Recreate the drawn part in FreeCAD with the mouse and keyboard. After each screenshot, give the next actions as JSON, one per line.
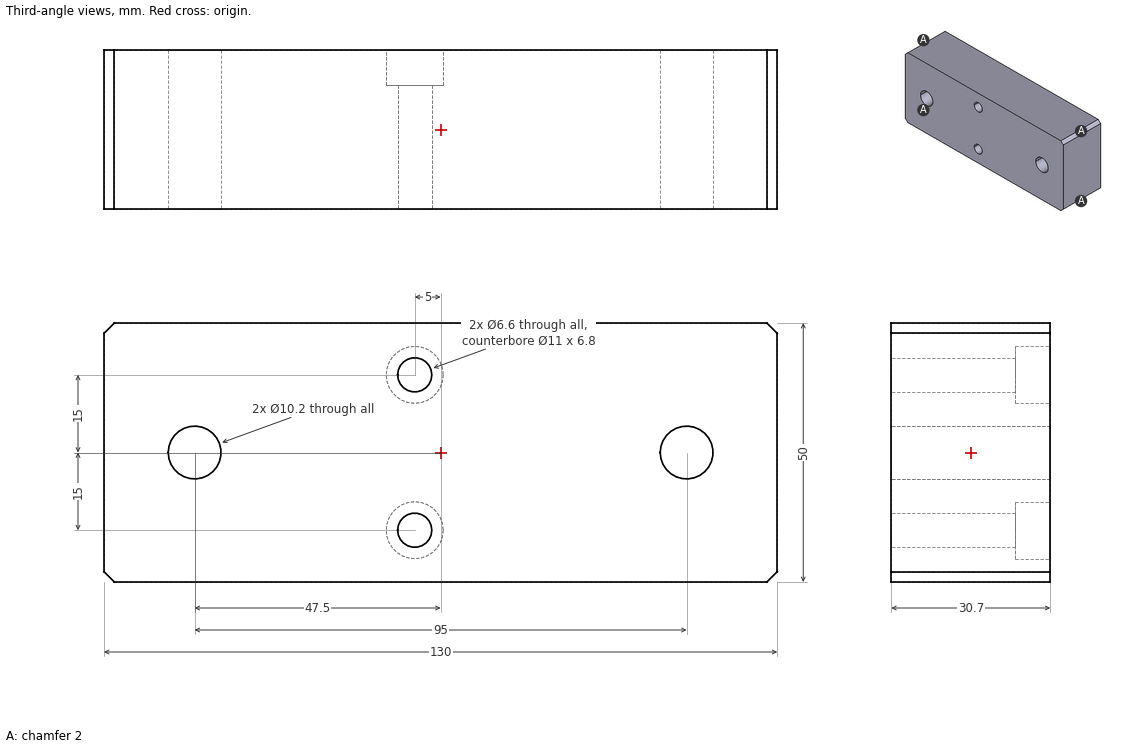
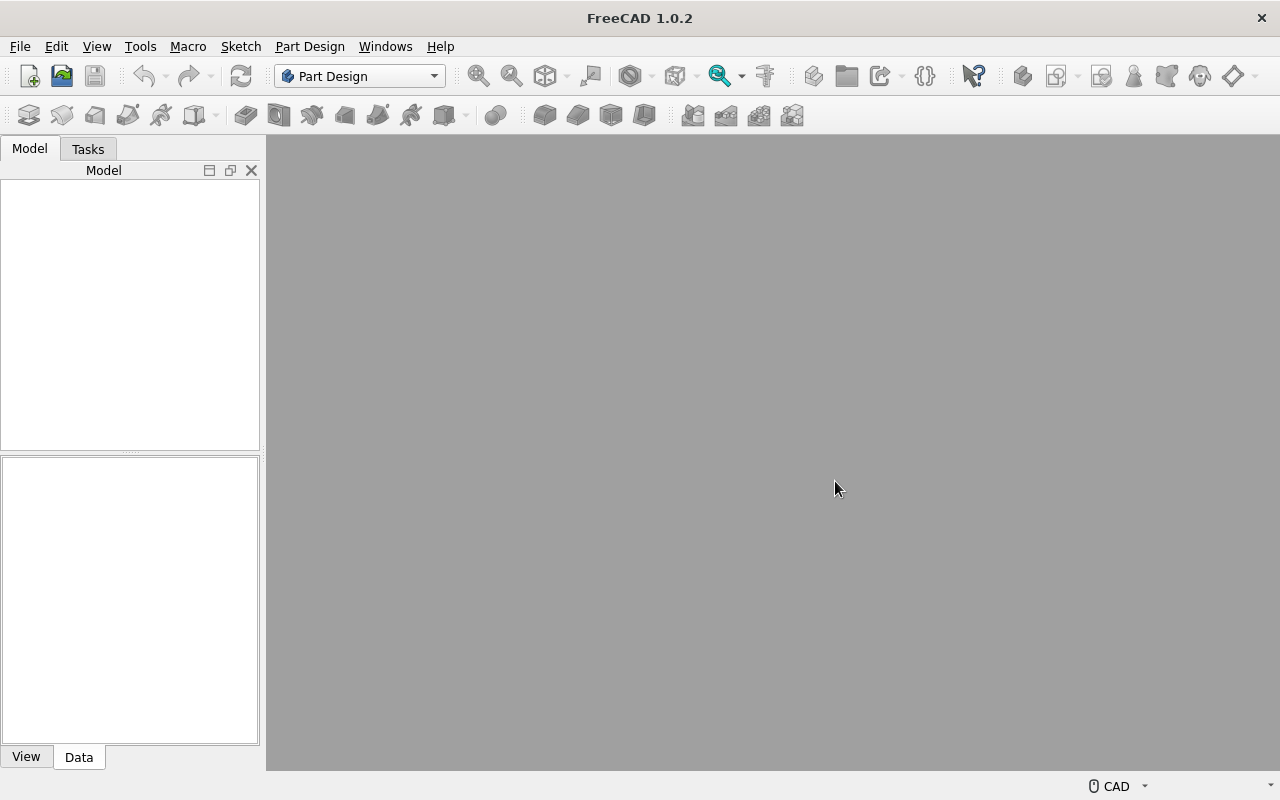
{"action": "left_click", "coordinate": [29, 76]}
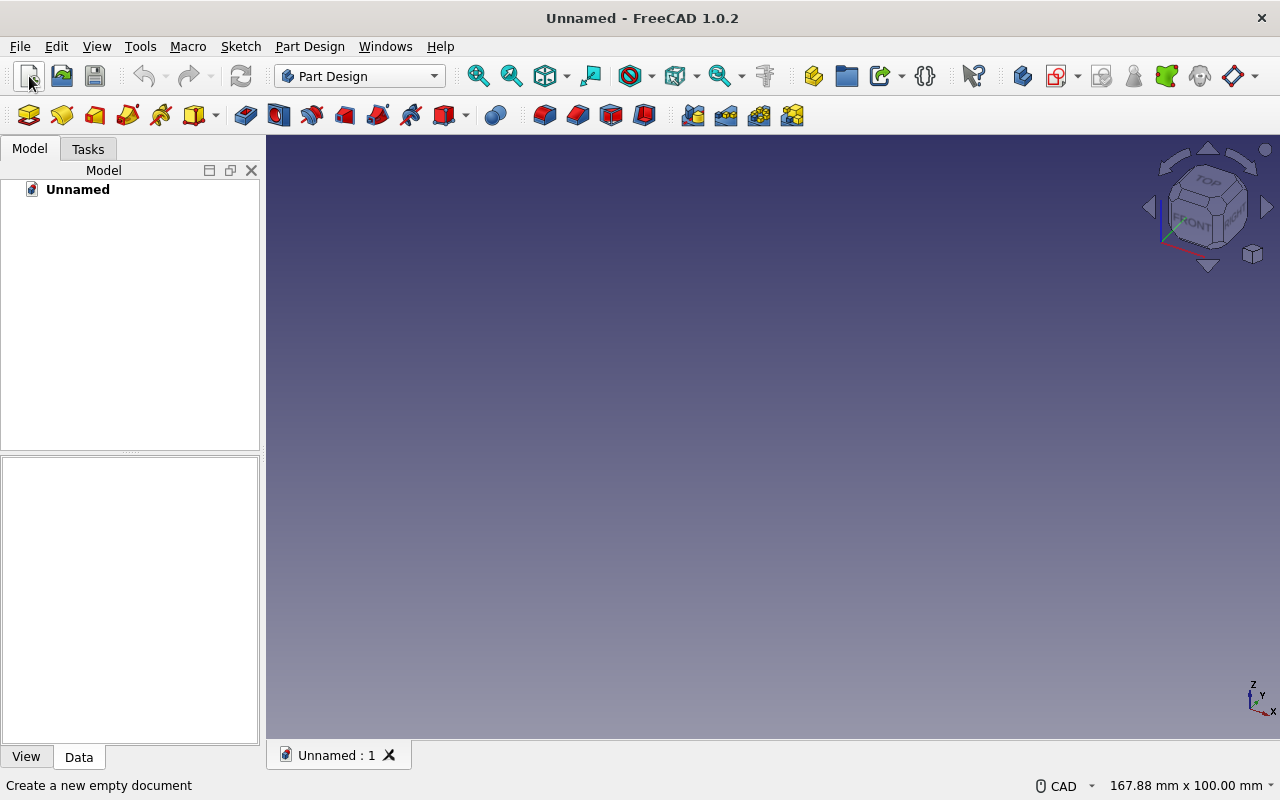
{"action": "left_click", "coordinate": [1056, 76]}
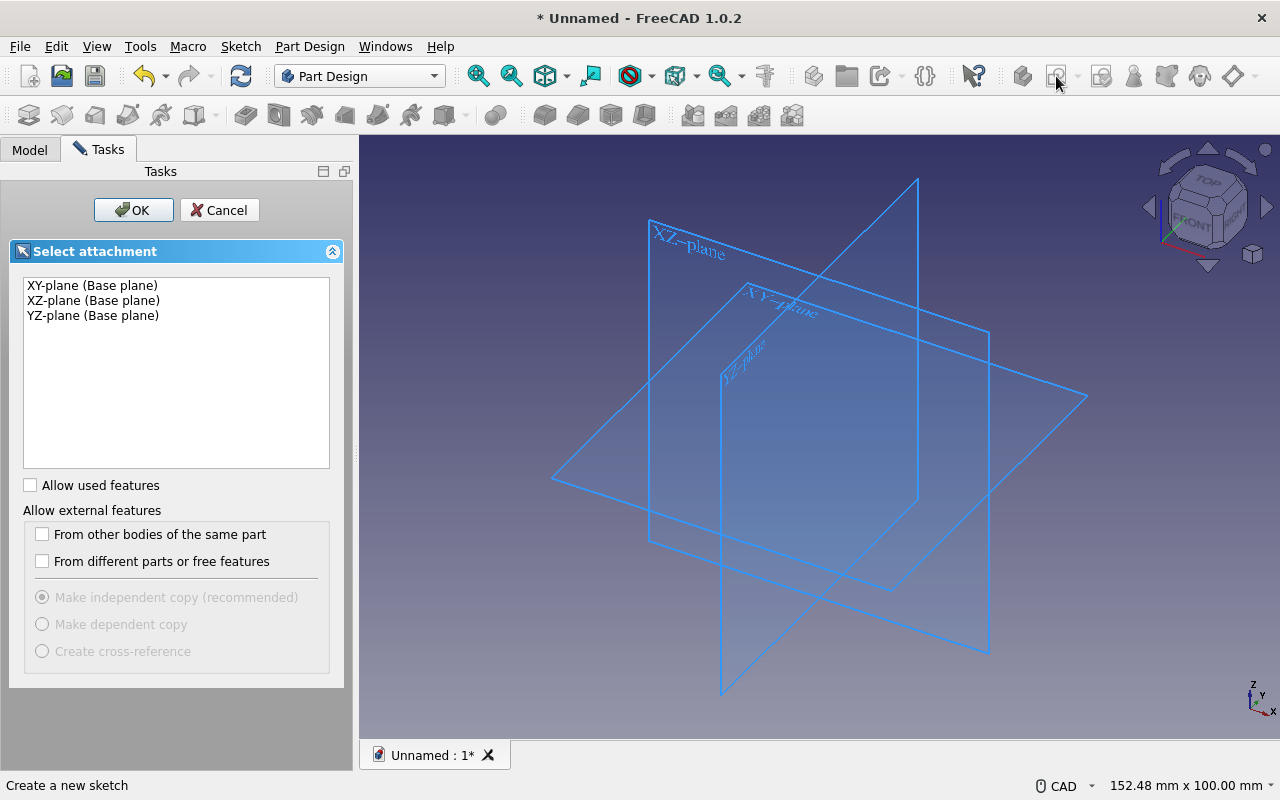
{"action": "left_click", "coordinate": [84, 300]}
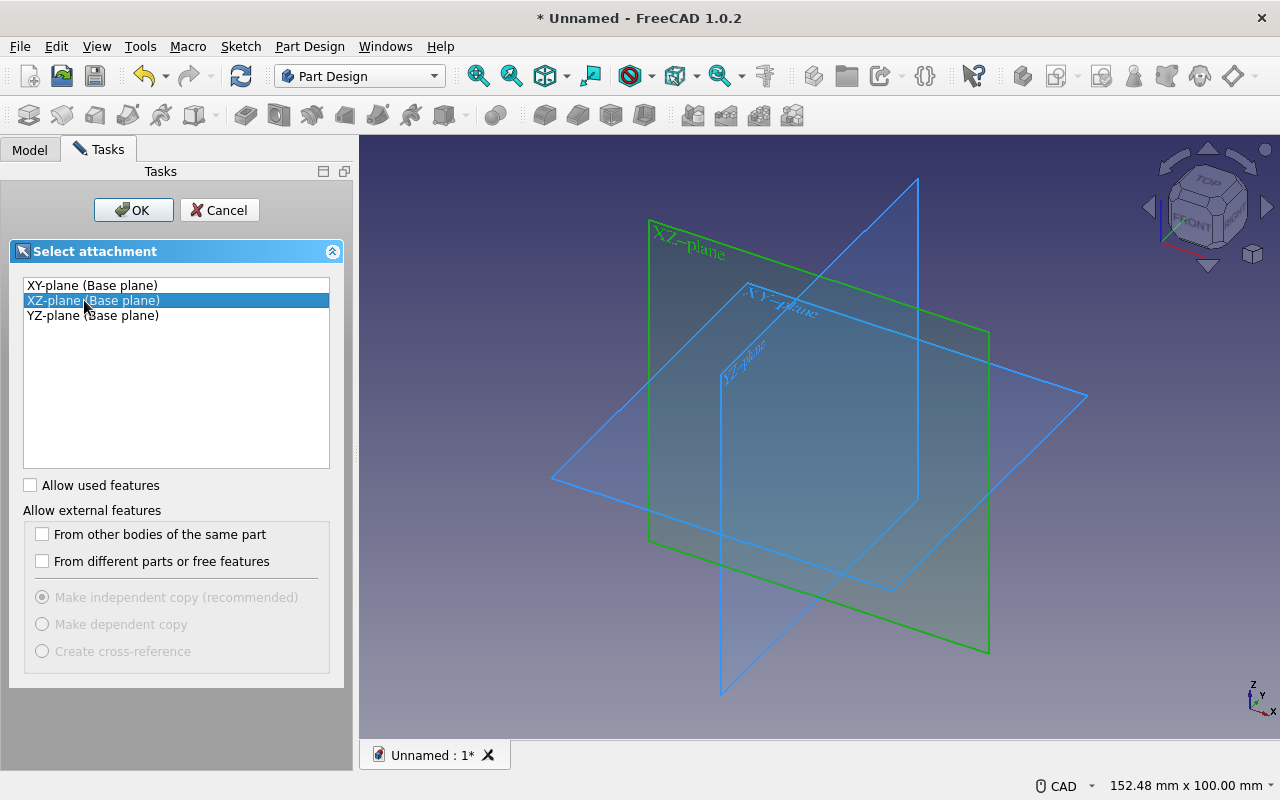
{"action": "left_click", "coordinate": [134, 210]}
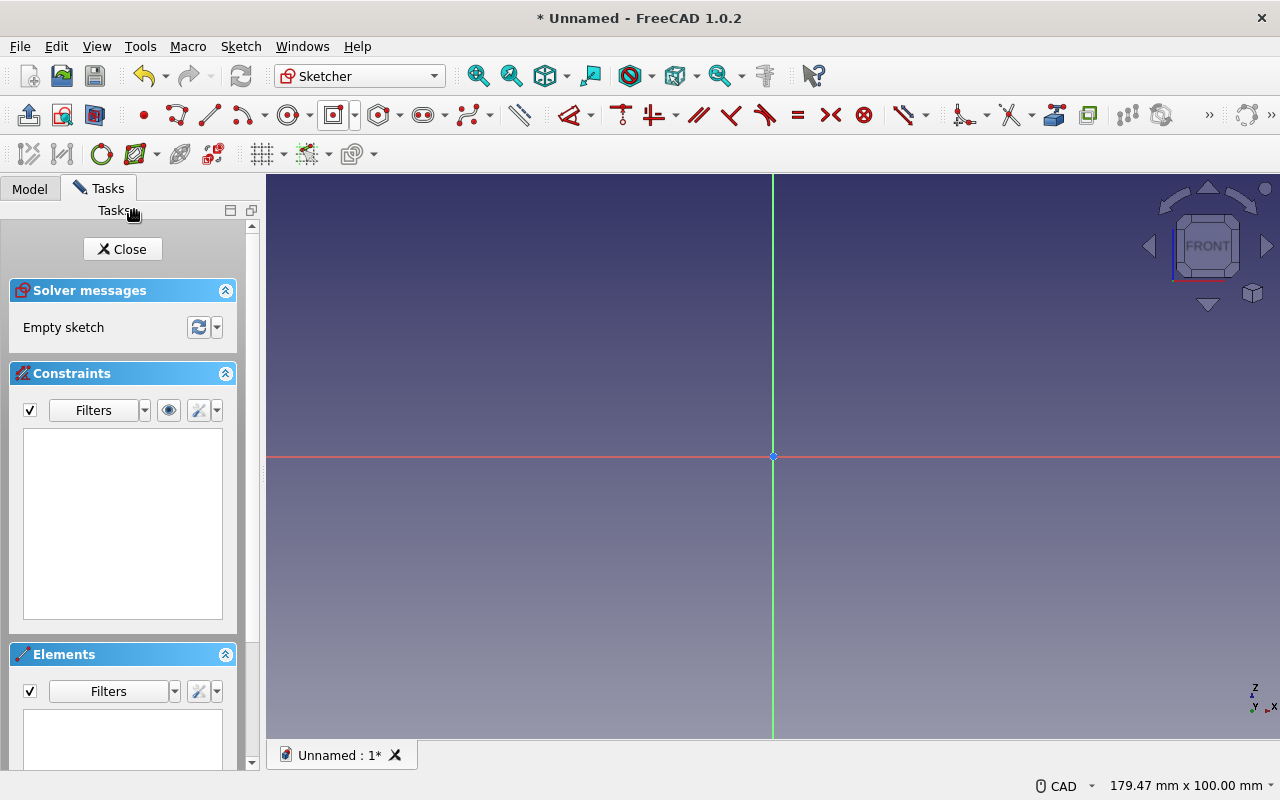
{"action": "scroll", "coordinate": [395, 456], "scroll_direction": "down", "scroll_amount": 1}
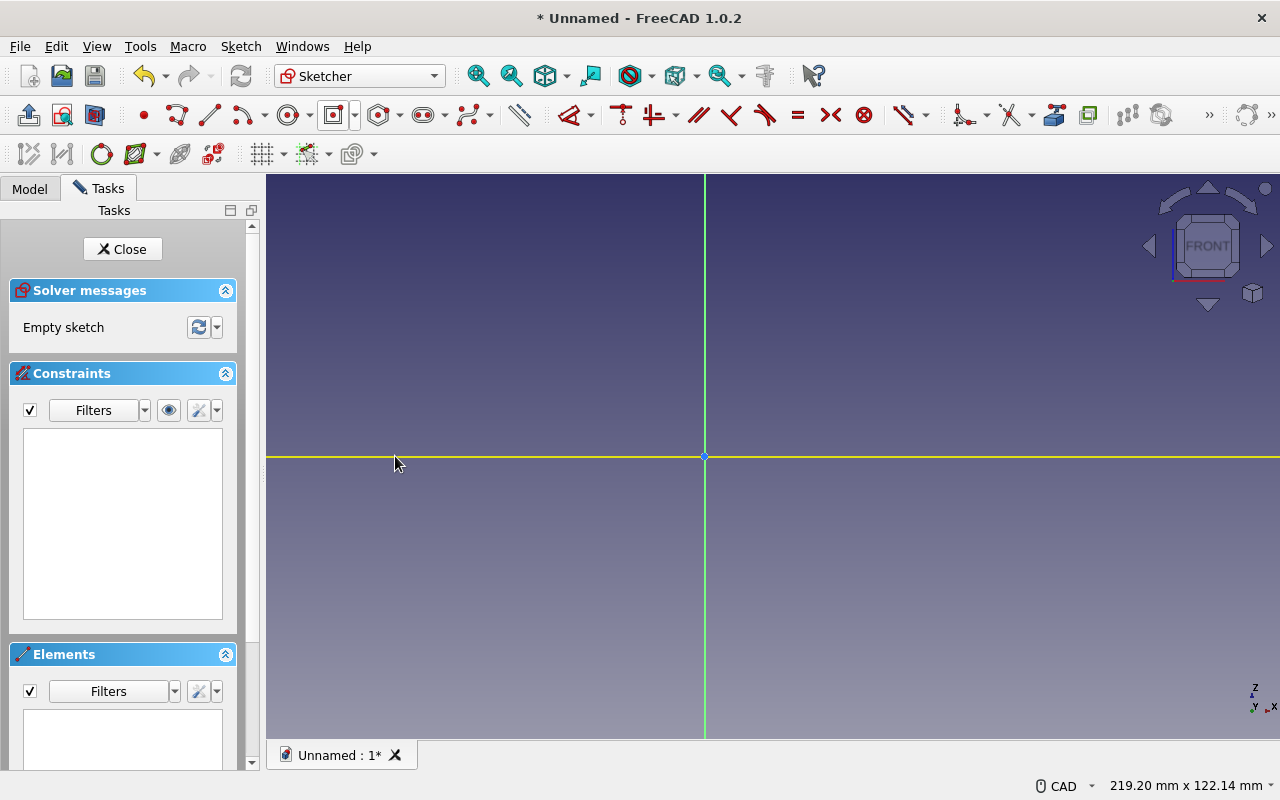
{"action": "key", "text": "g v"}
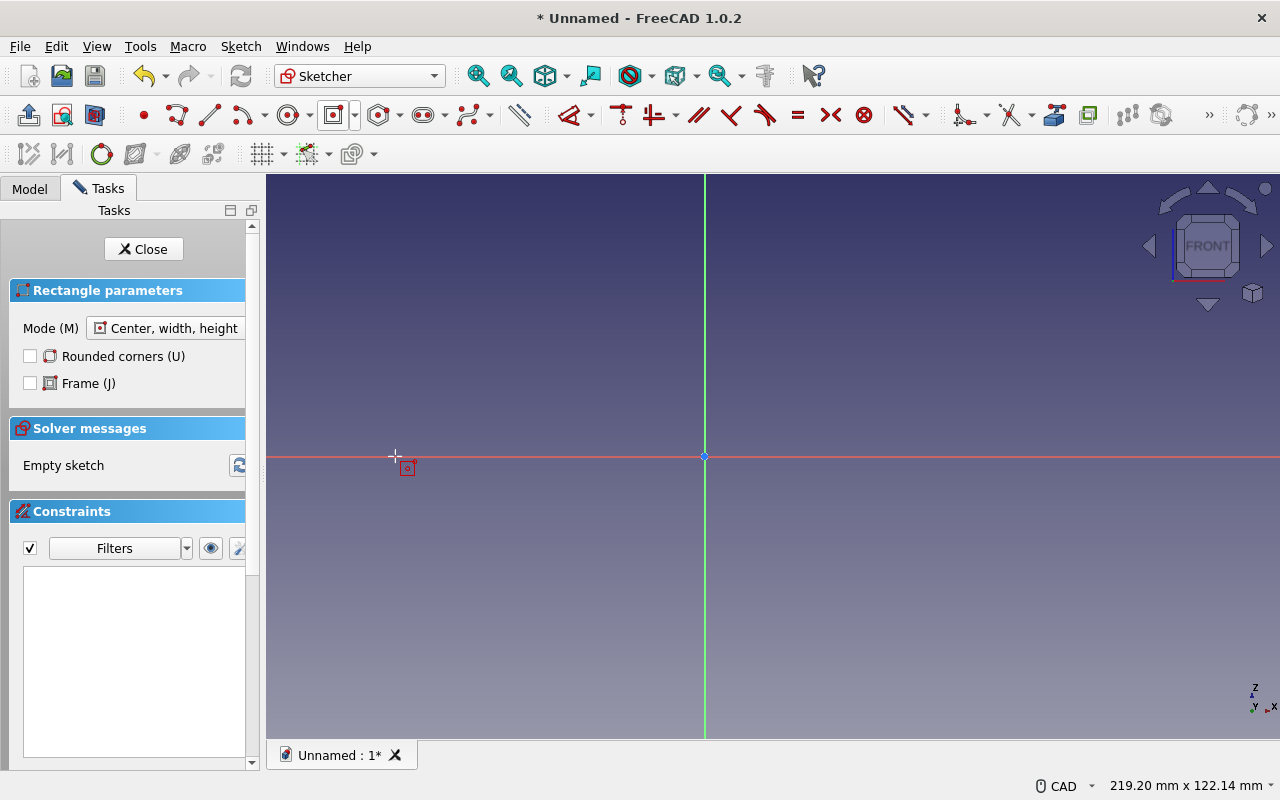
{"action": "left_click", "coordinate": [705, 456]}
{"action": "left_click", "coordinate": [1005, 341]}
{"action": "key", "text": "Escape"}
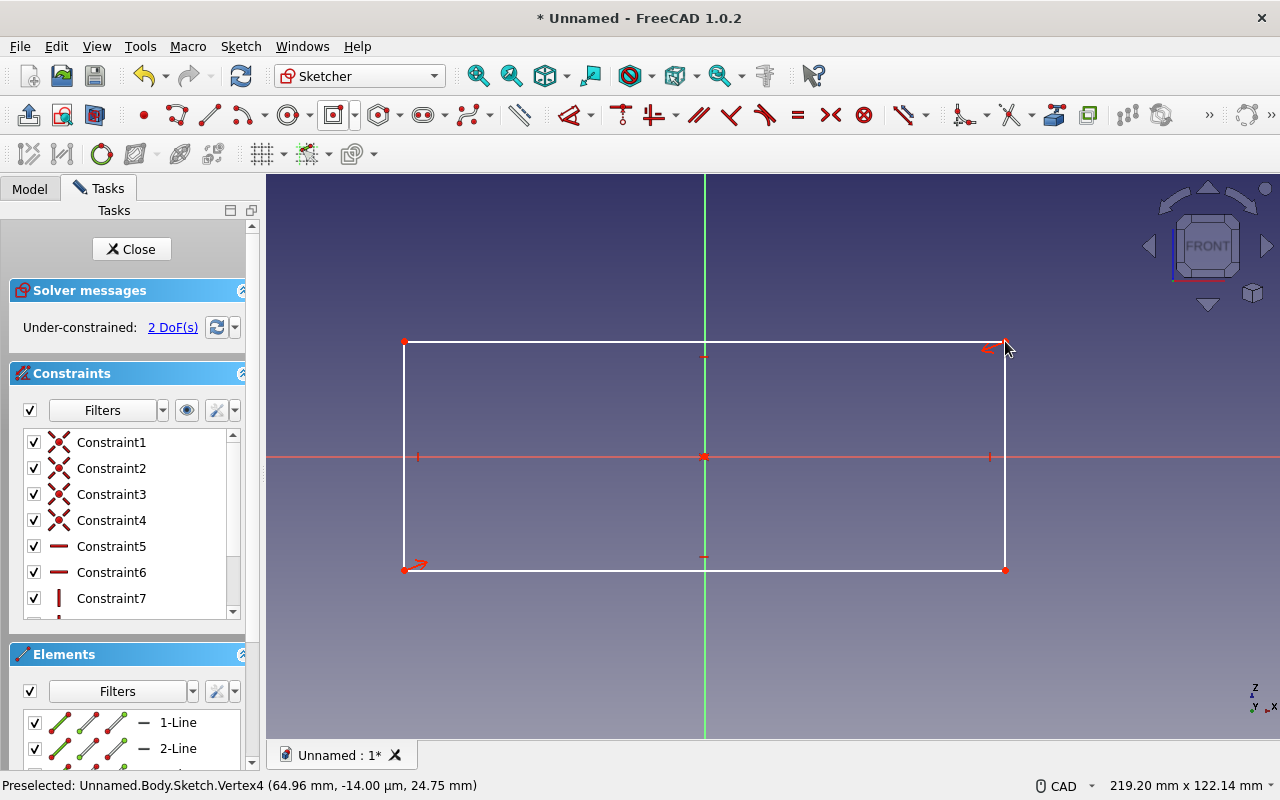
{"action": "left_click", "coordinate": [1005, 502]}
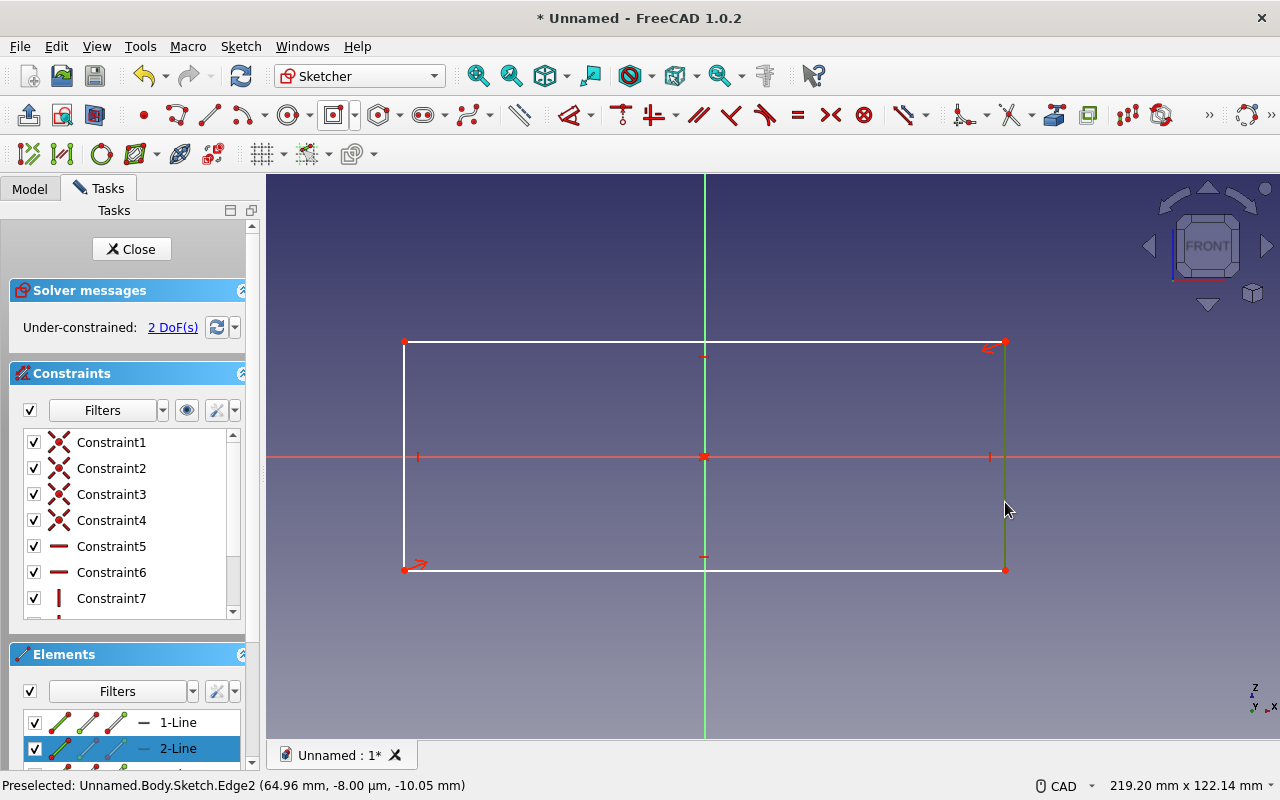
{"action": "left_click", "coordinate": [590, 116]}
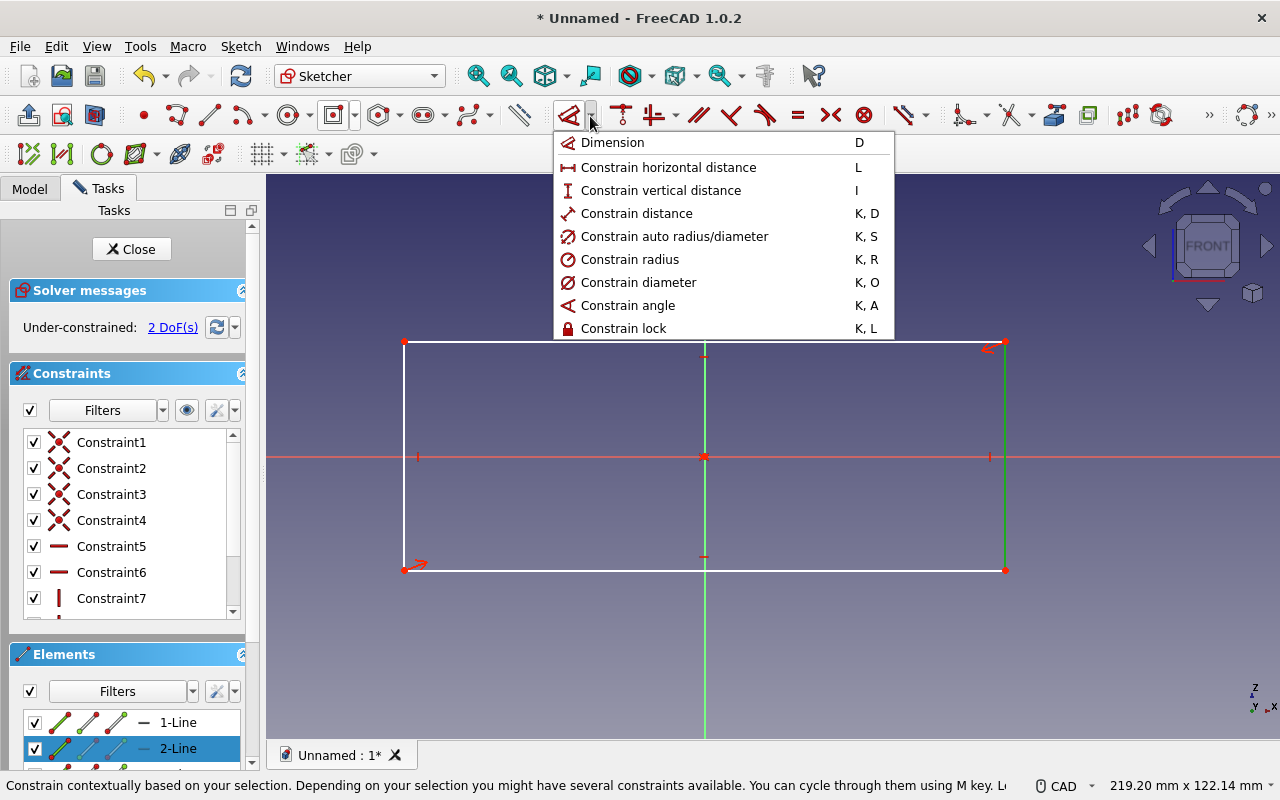
{"action": "left_click", "coordinate": [724, 190]}